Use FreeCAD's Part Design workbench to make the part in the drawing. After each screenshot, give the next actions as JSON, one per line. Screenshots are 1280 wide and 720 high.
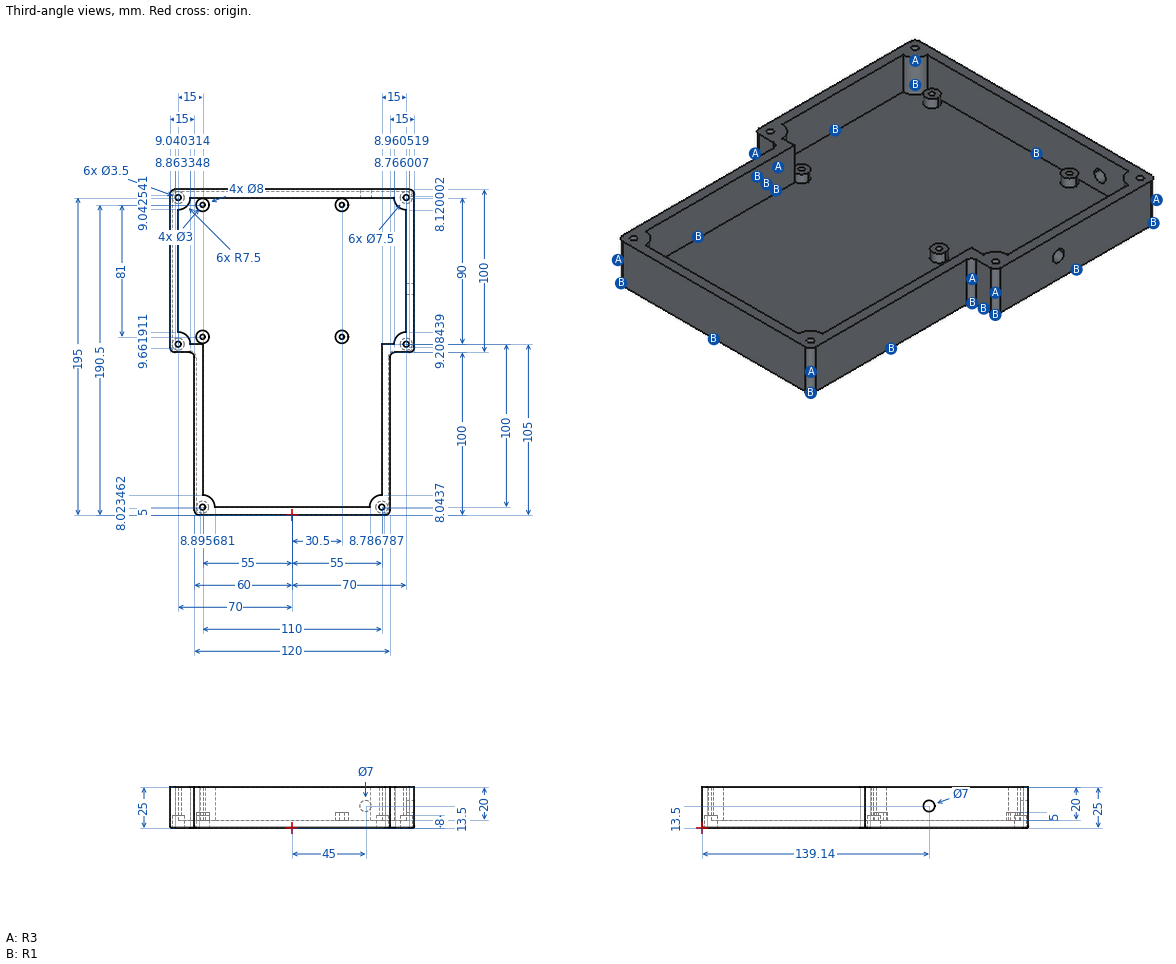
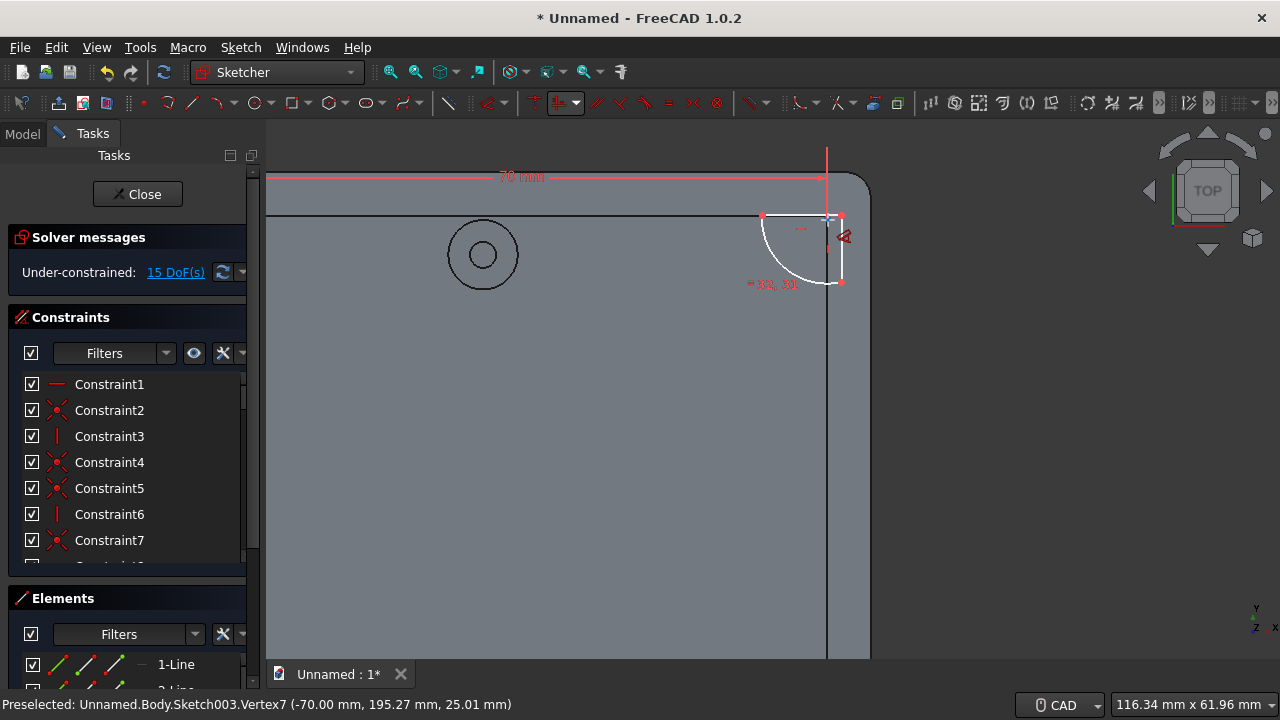
{"action": "left_click", "coordinate": [827, 218]}
{"action": "left_click", "coordinate": [861, 425]}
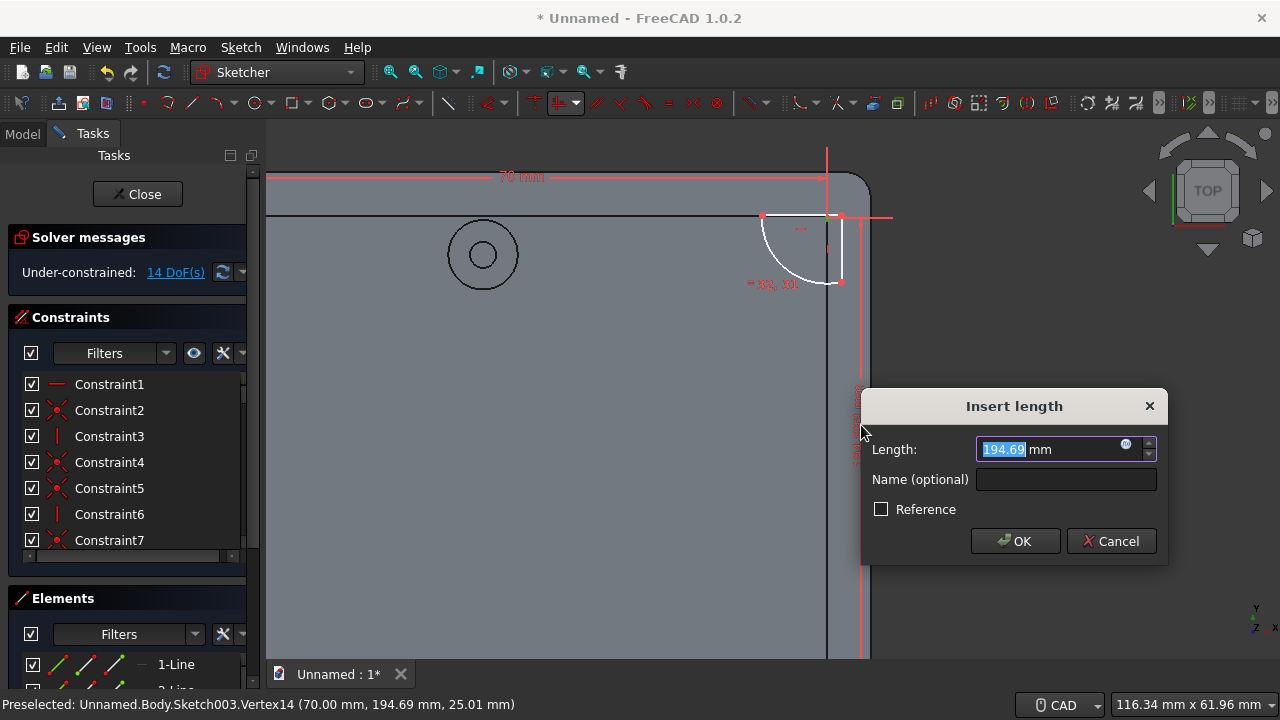
{"action": "type", "text": "195"}
{"action": "key", "text": "Return"}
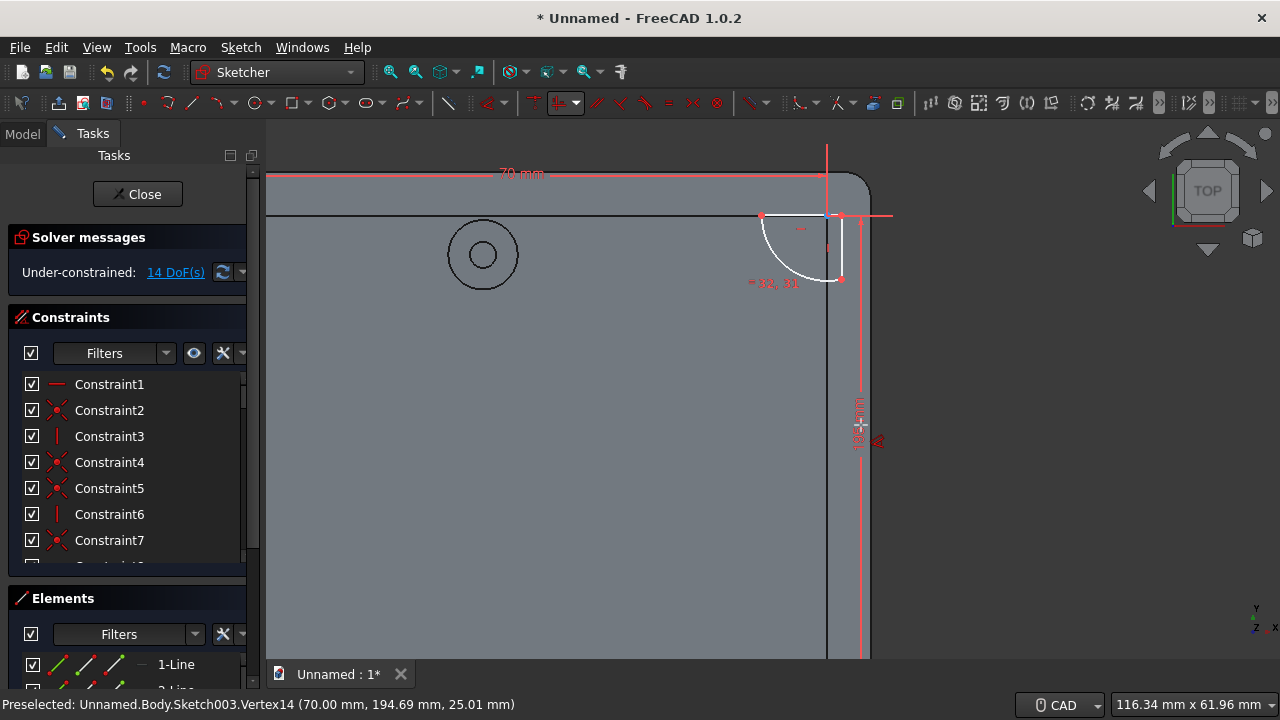
{"action": "scroll", "coordinate": [828, 220], "scroll_direction": "down", "scroll_amount": 8}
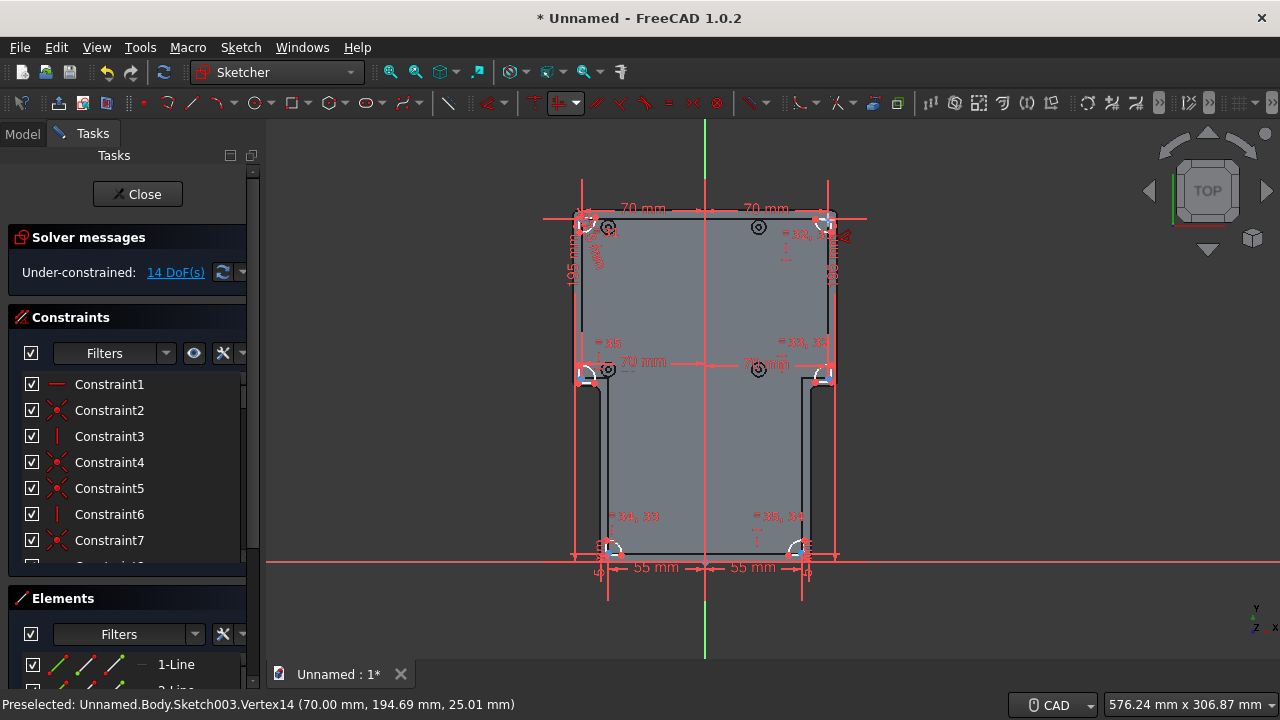
{"action": "scroll", "coordinate": [828, 378], "scroll_direction": "up", "scroll_amount": 5}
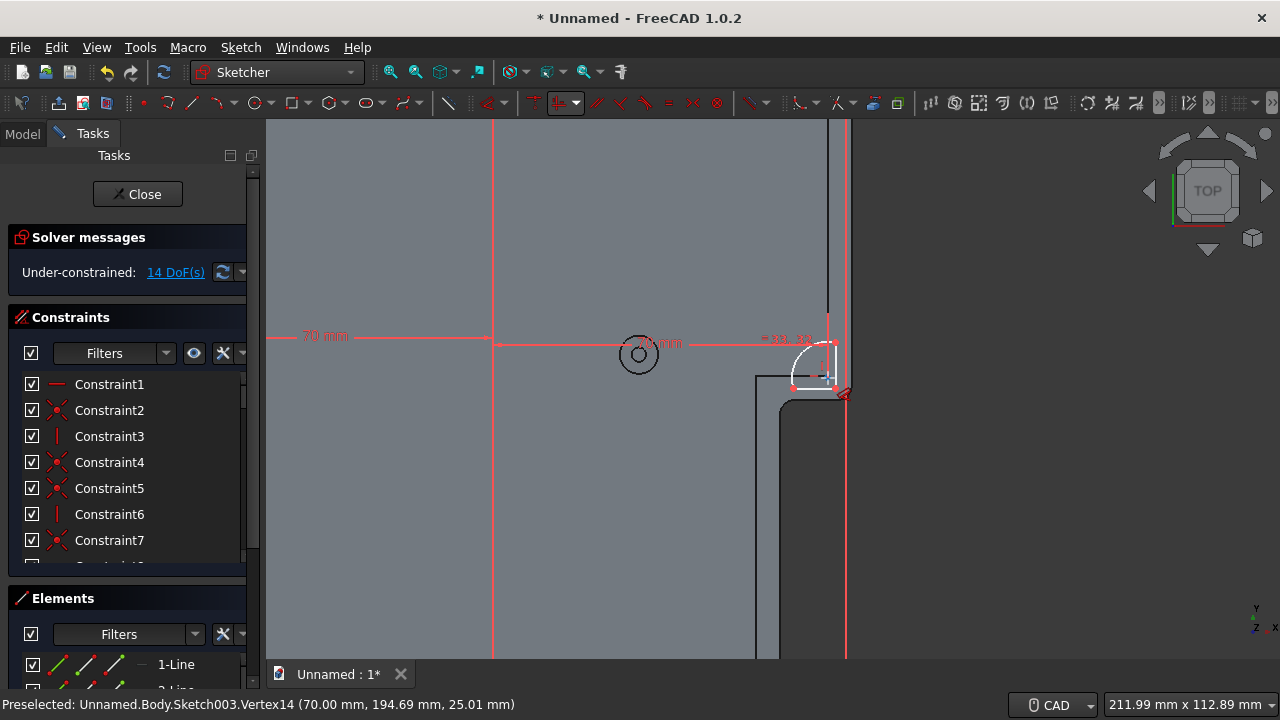
{"action": "left_click", "coordinate": [828, 378]}
{"action": "left_click", "coordinate": [862, 504]}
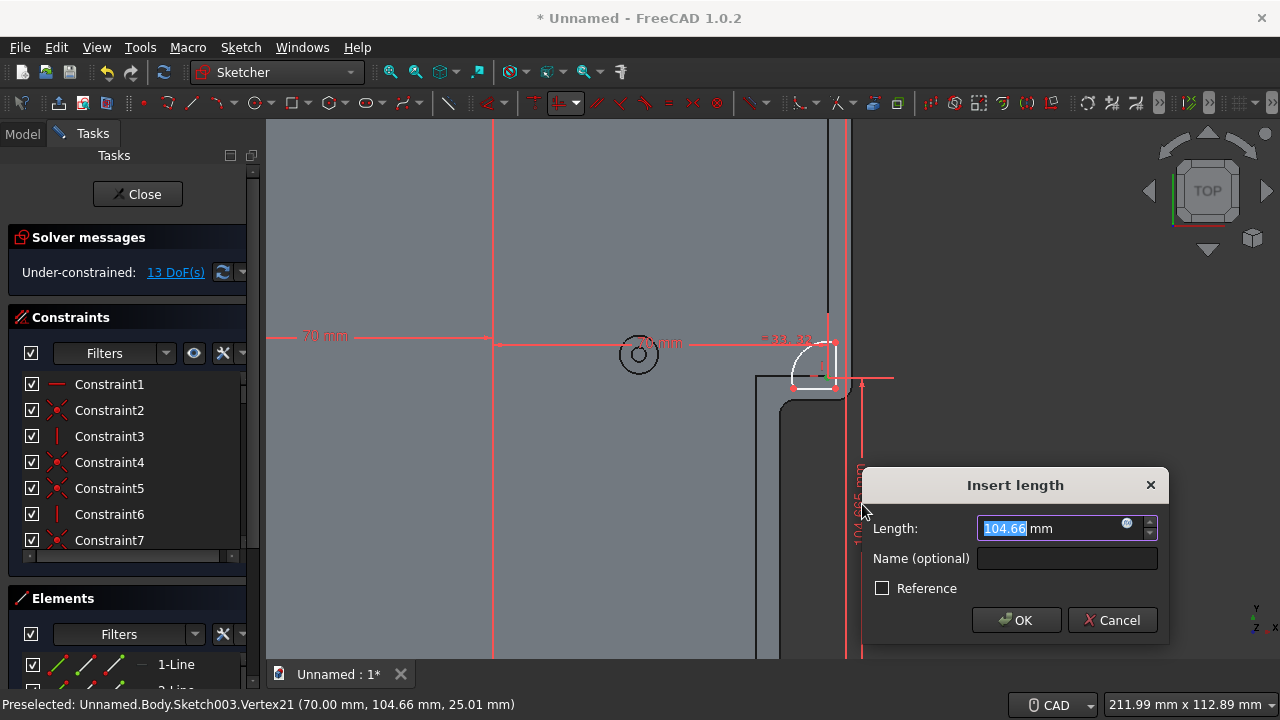
{"action": "type", "text": "105"}
{"action": "key", "text": "Return"}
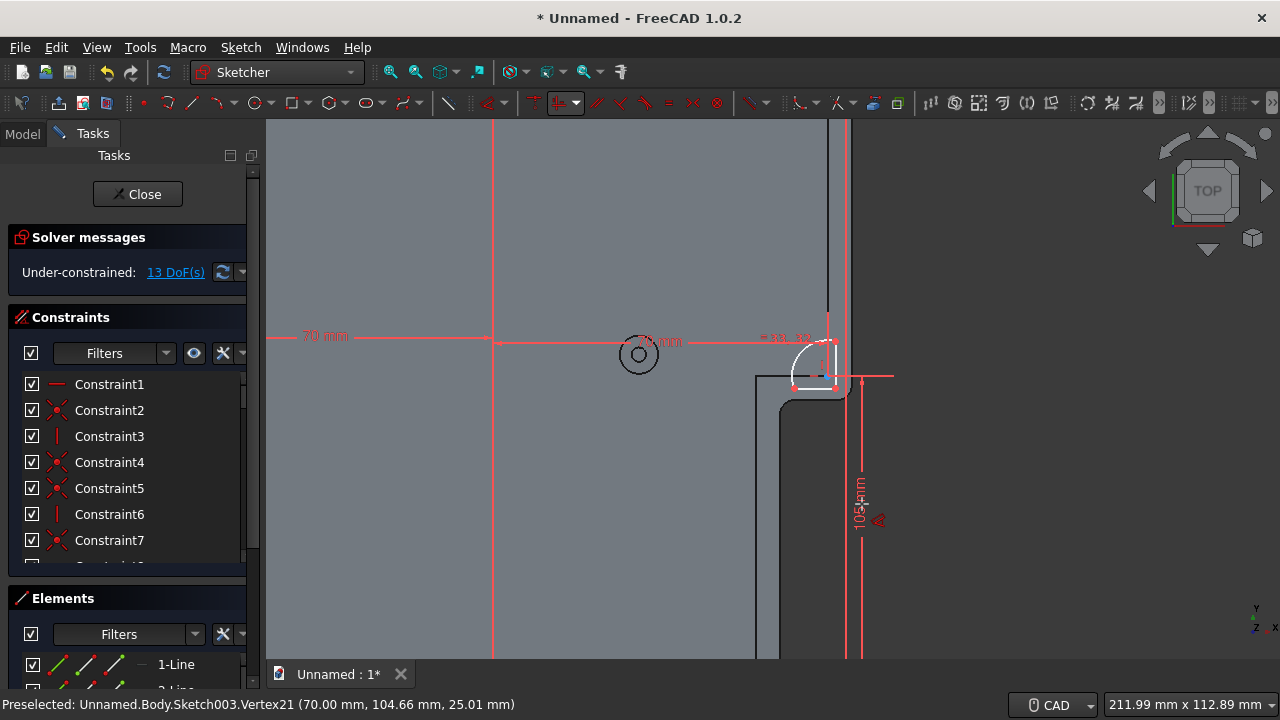
{"action": "scroll", "coordinate": [828, 378], "scroll_direction": "down", "scroll_amount": 5}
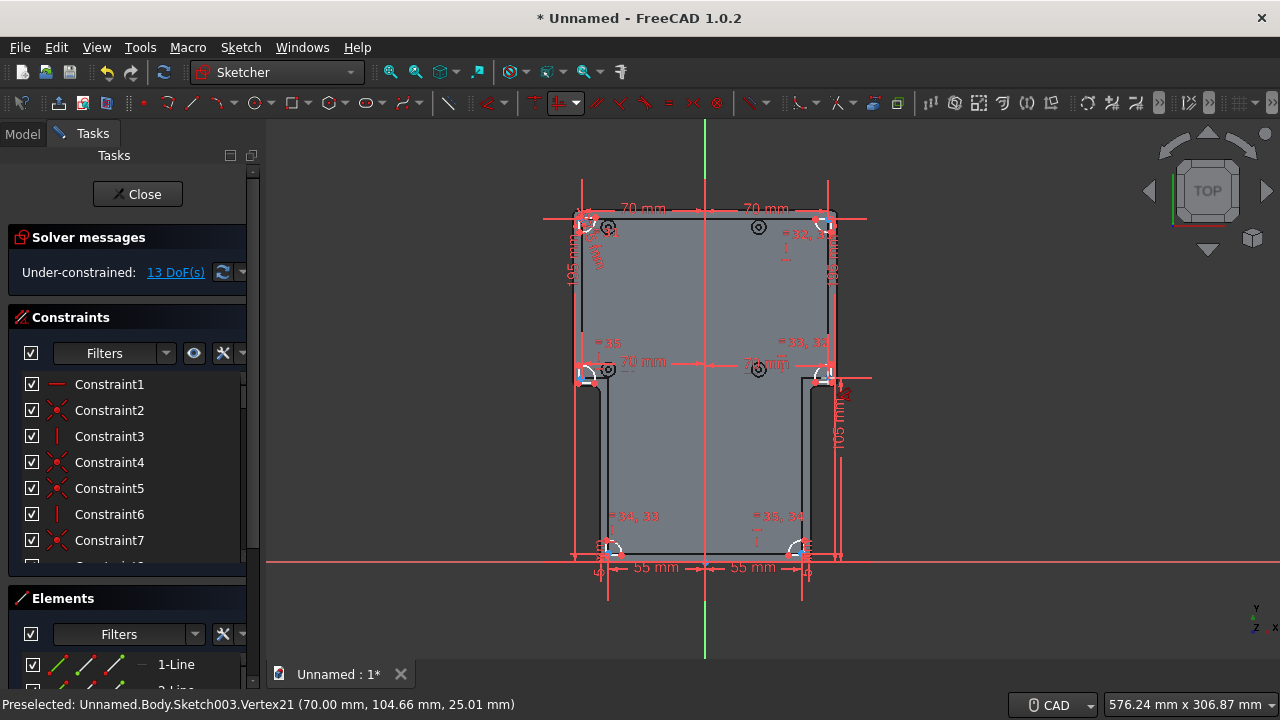
{"action": "scroll", "coordinate": [582, 379], "scroll_direction": "up", "scroll_amount": 5}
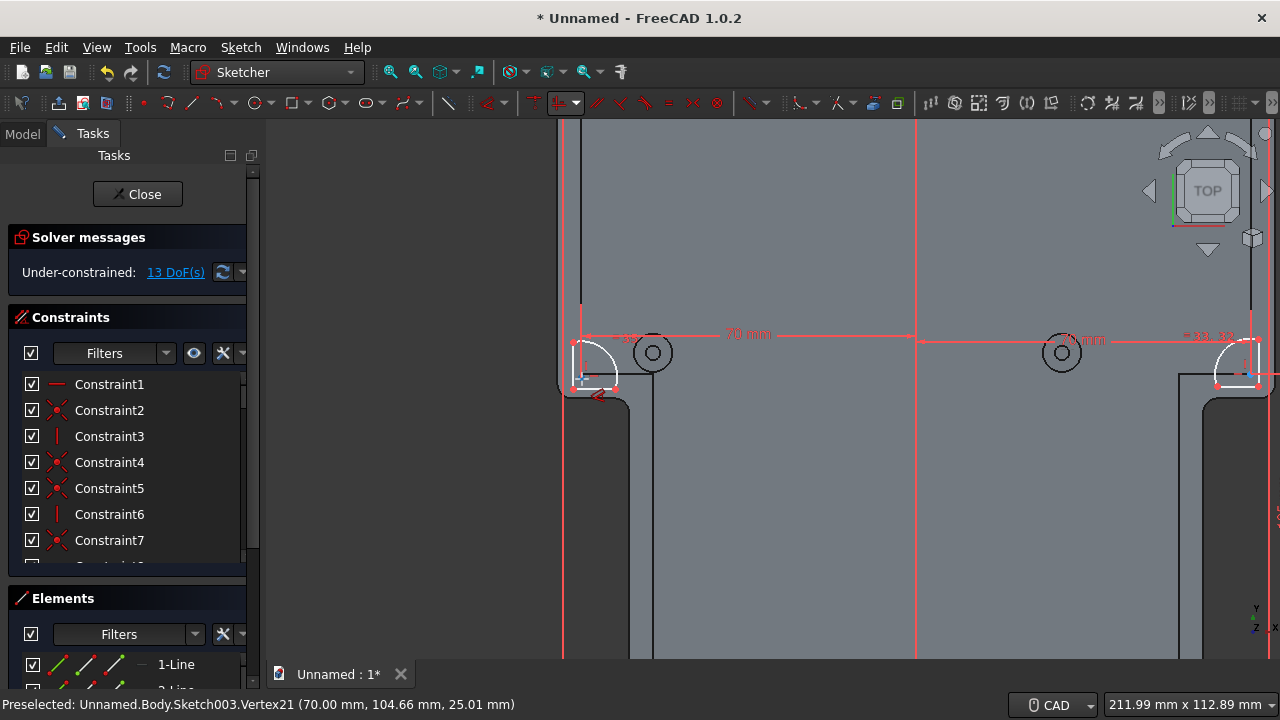
{"action": "left_click", "coordinate": [581, 377]}
{"action": "left_click", "coordinate": [547, 504]}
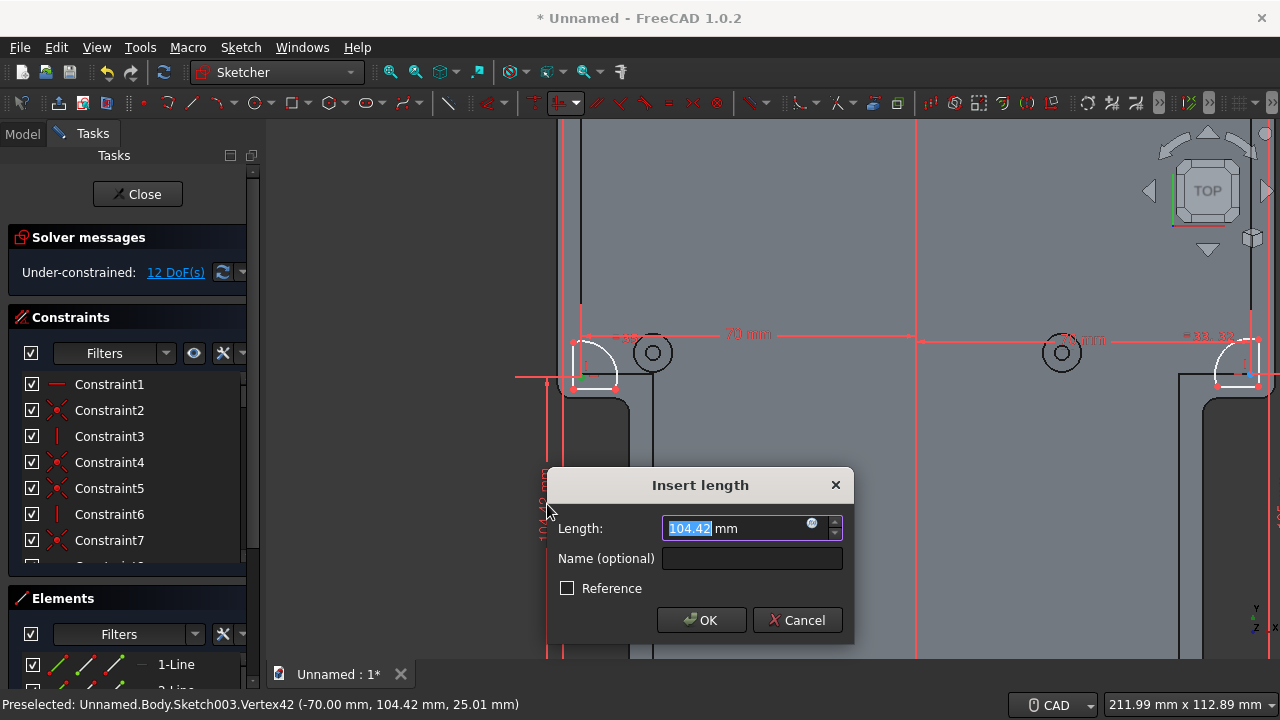
{"action": "type", "text": "105"}
{"action": "key", "text": "Return"}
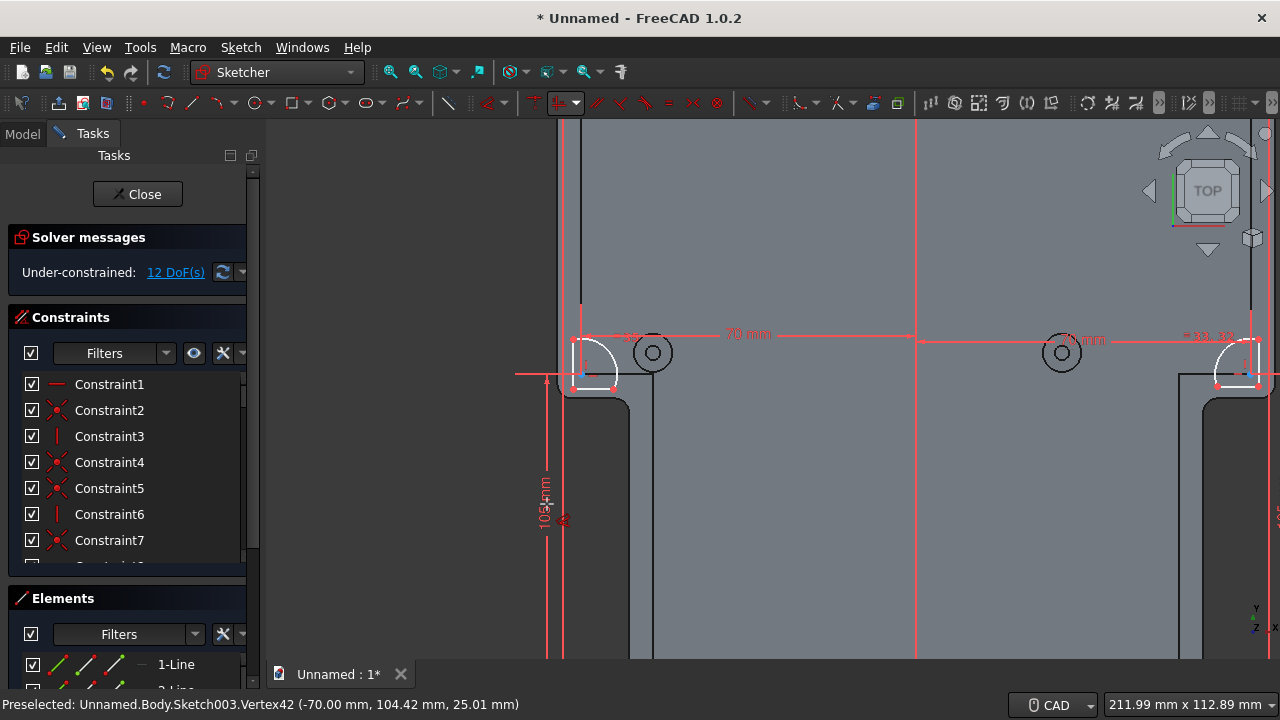
{"action": "scroll", "coordinate": [582, 379], "scroll_direction": "down", "scroll_amount": 5}